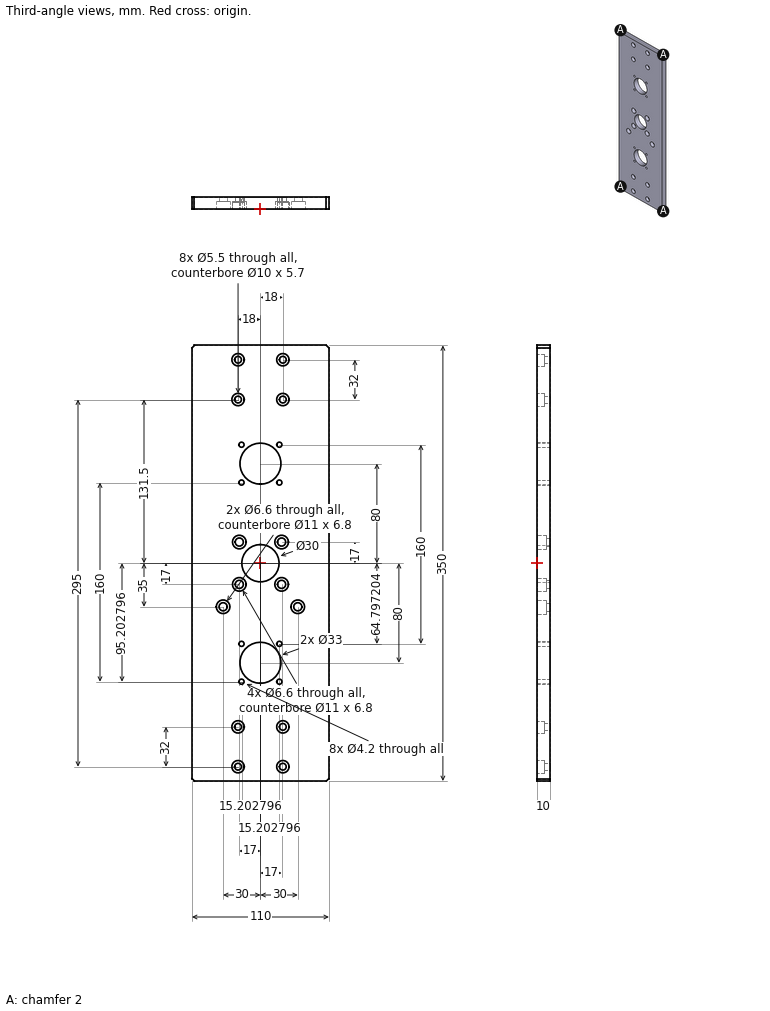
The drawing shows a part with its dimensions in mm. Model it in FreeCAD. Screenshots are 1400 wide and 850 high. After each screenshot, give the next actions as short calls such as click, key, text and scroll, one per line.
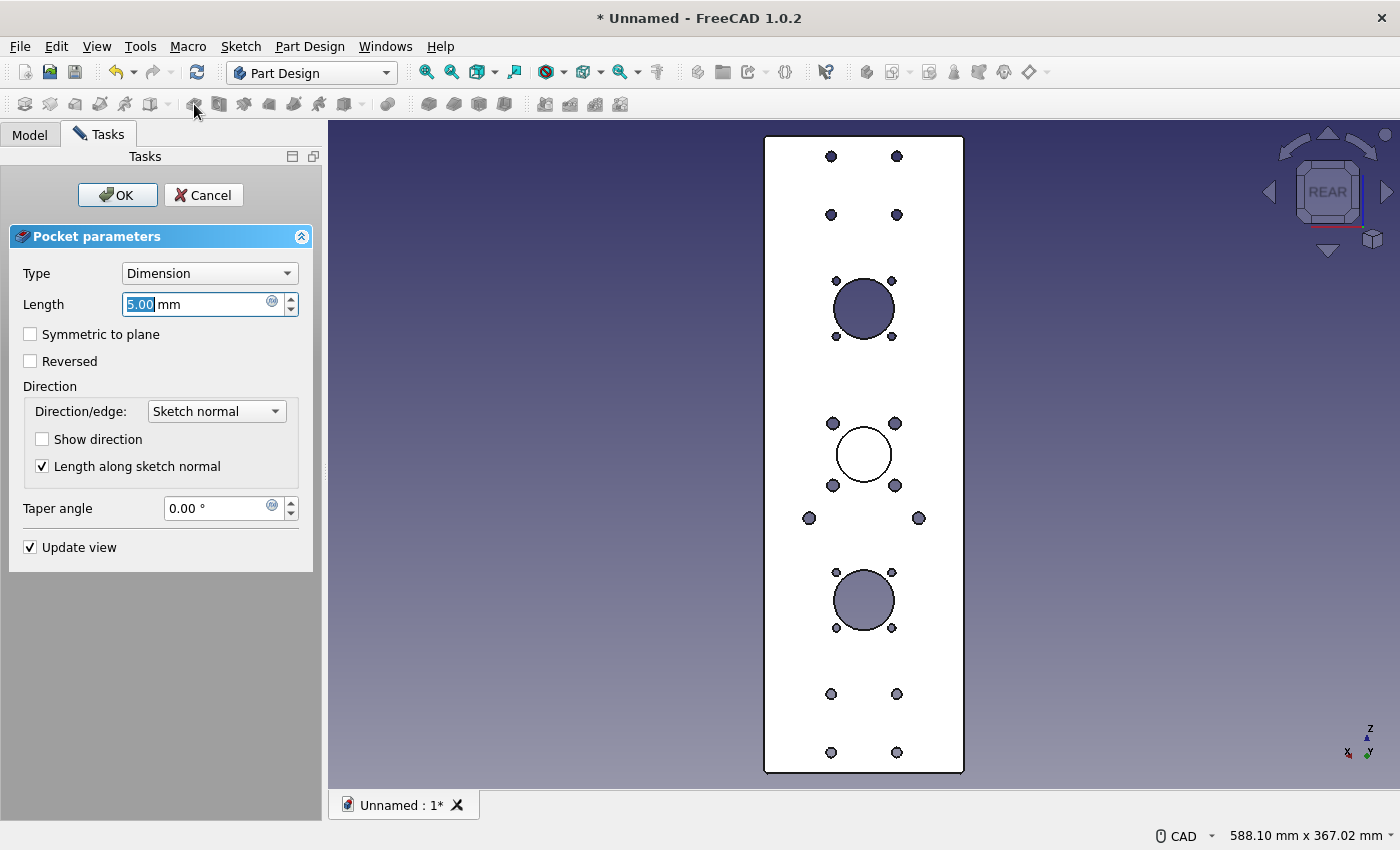
click(210, 274)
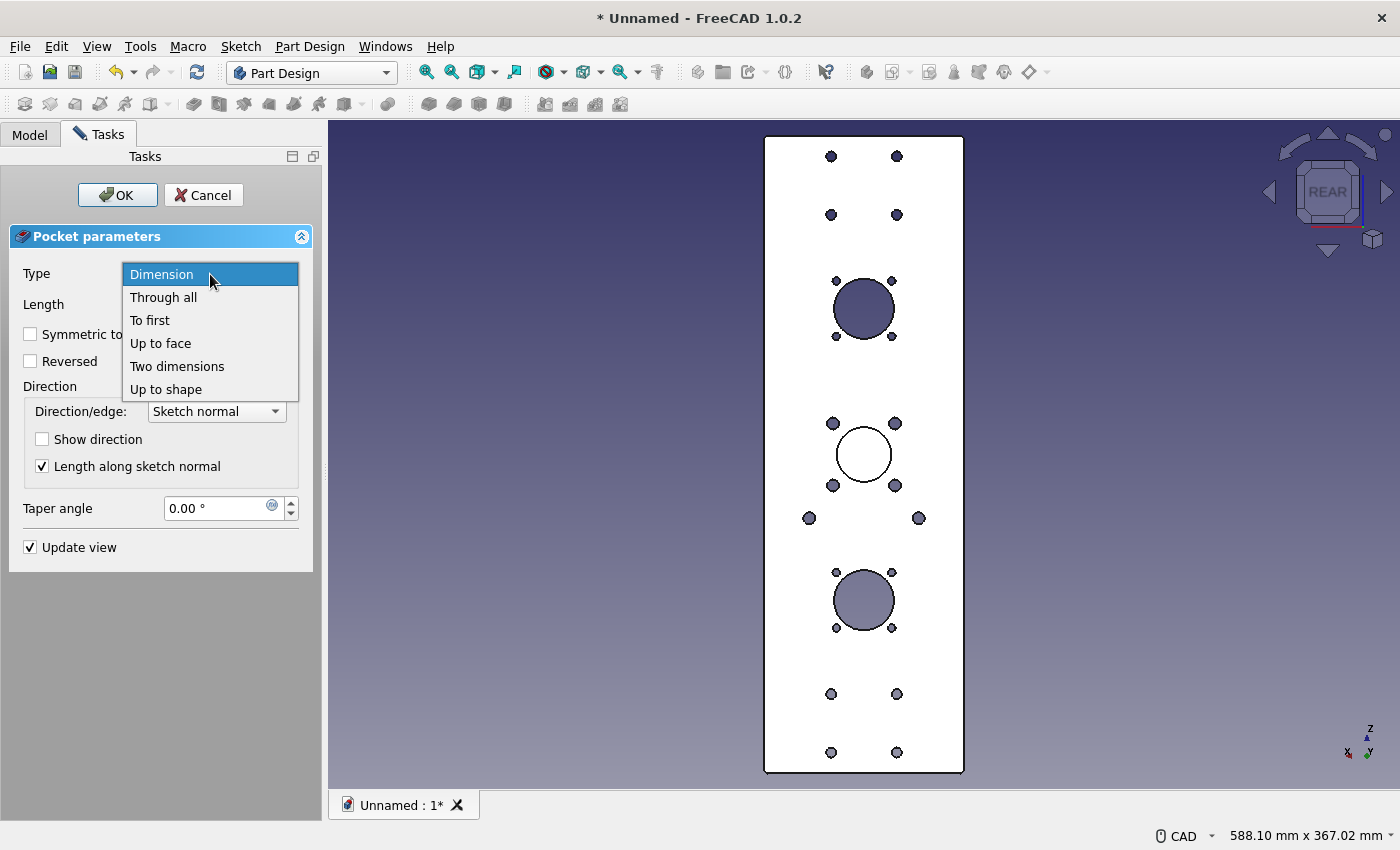
click(208, 298)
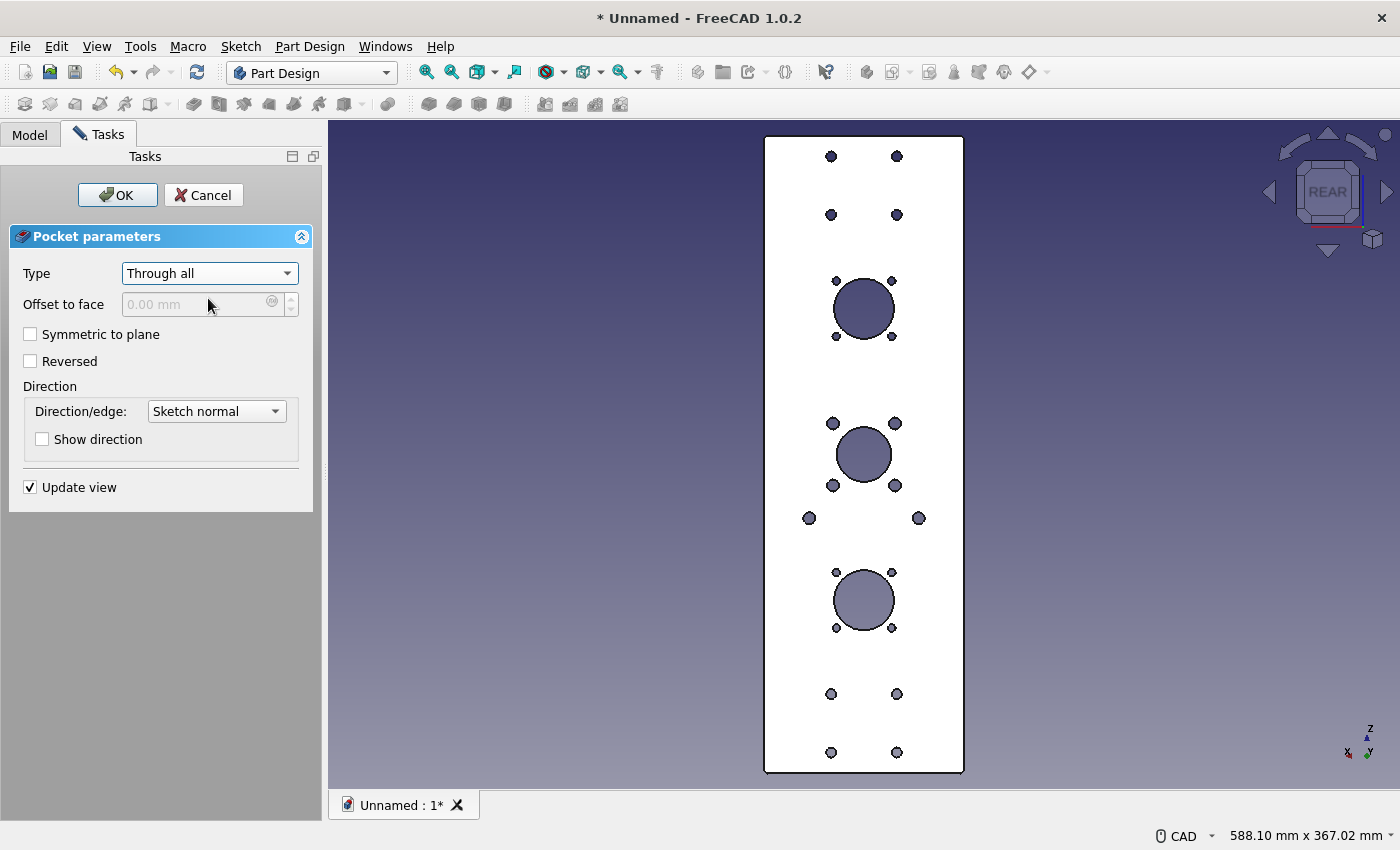
click(118, 195)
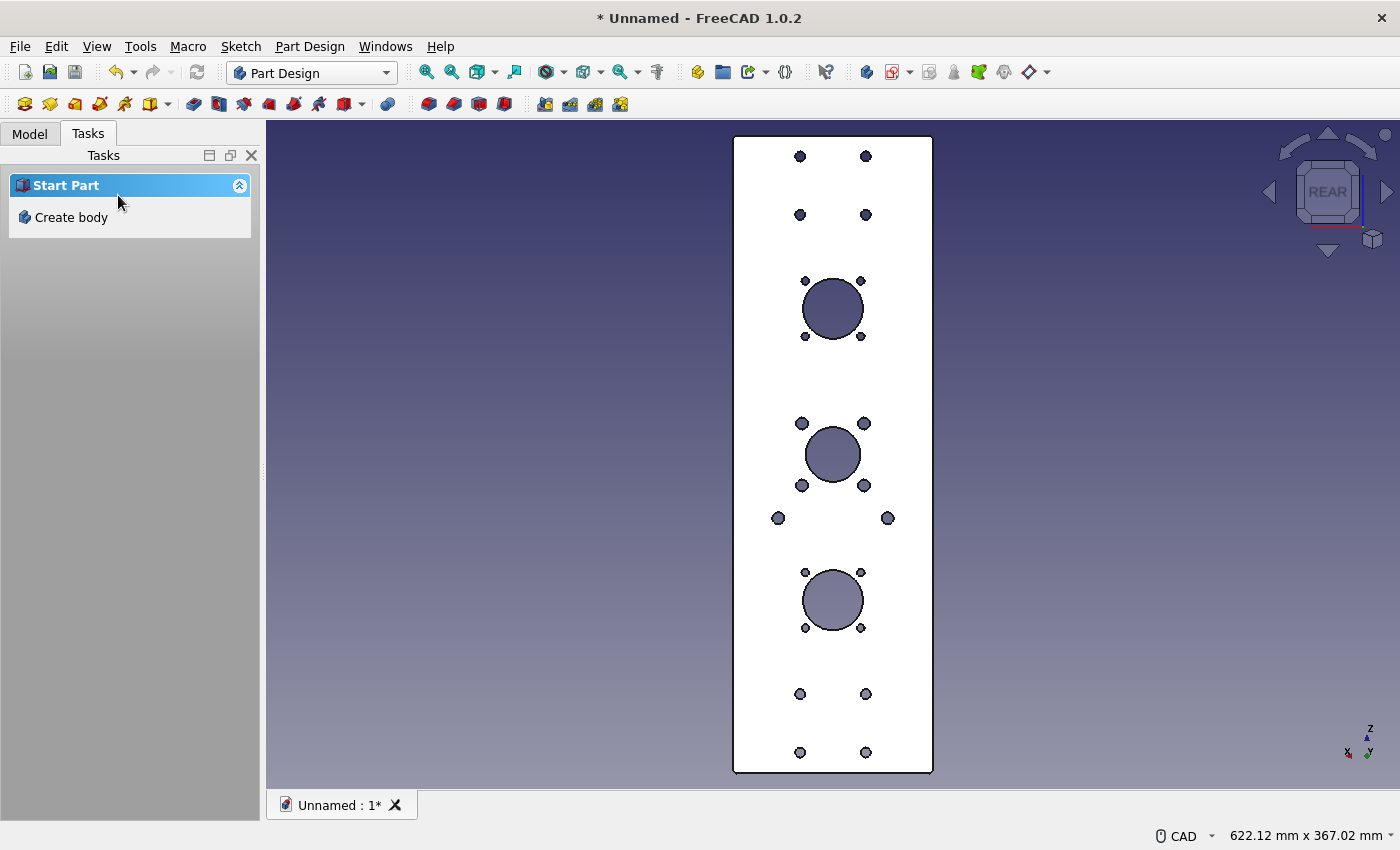
key(0)